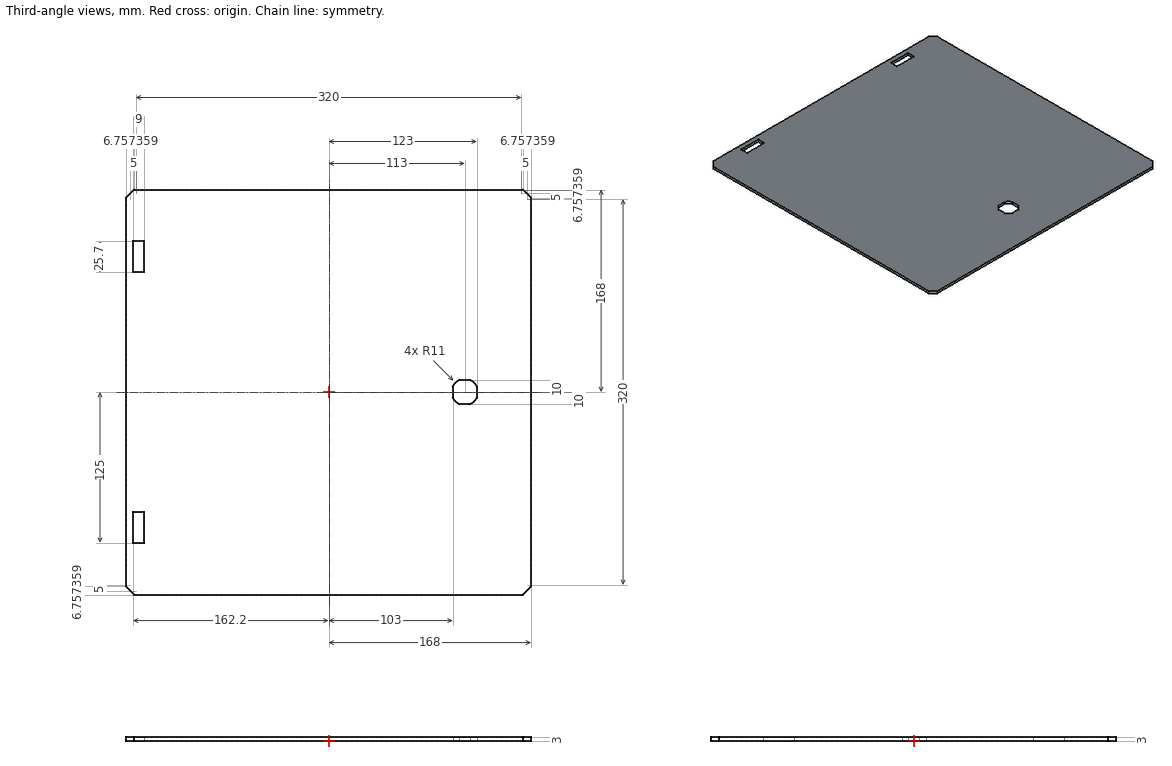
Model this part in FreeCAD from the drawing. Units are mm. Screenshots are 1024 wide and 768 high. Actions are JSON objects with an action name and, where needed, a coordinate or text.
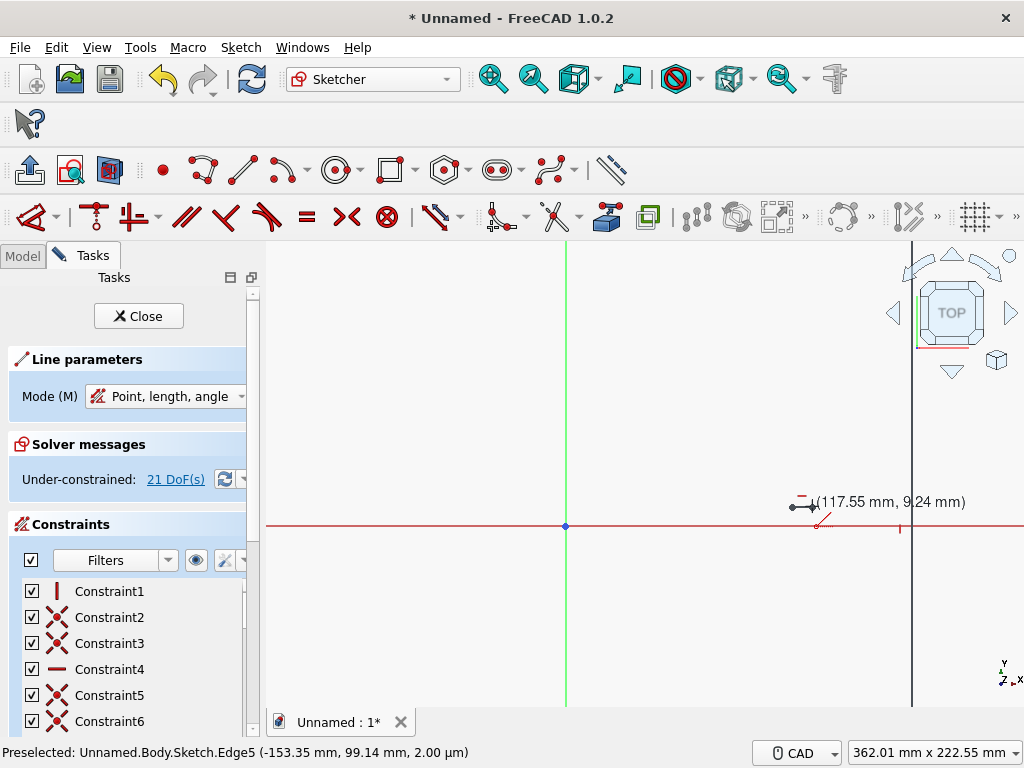
{"action": "scroll", "coordinate": [823, 517], "scroll_direction": "up", "scroll_amount": 3}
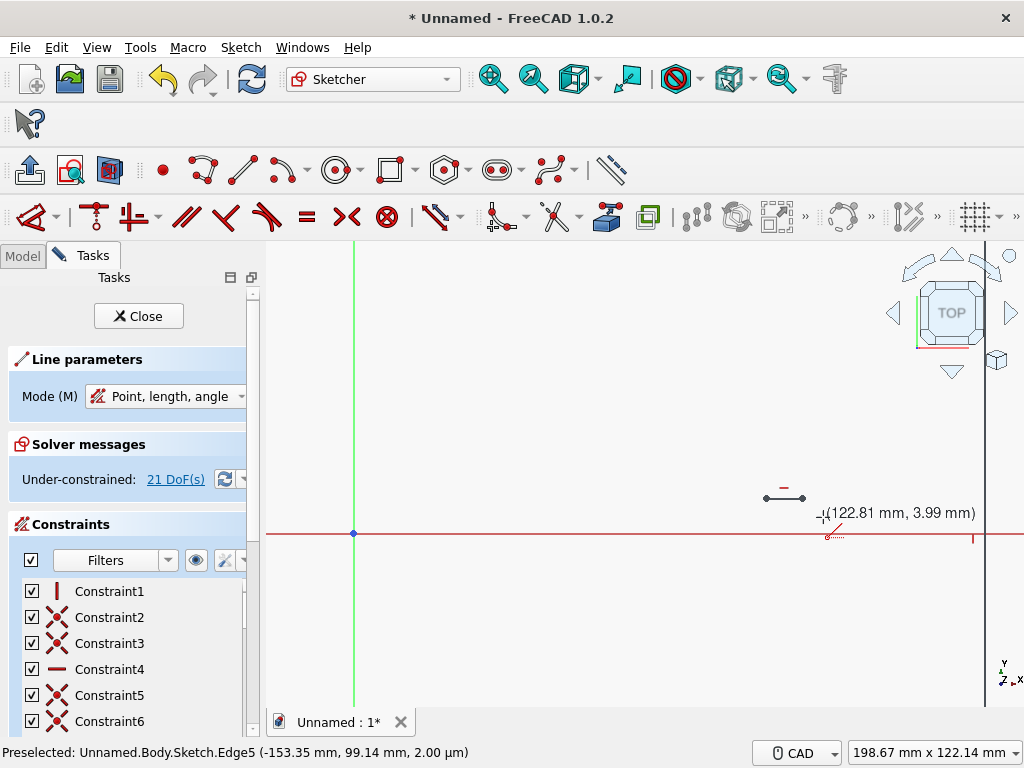
{"action": "left_click", "coordinate": [823, 516]}
{"action": "left_click", "coordinate": [823, 551]}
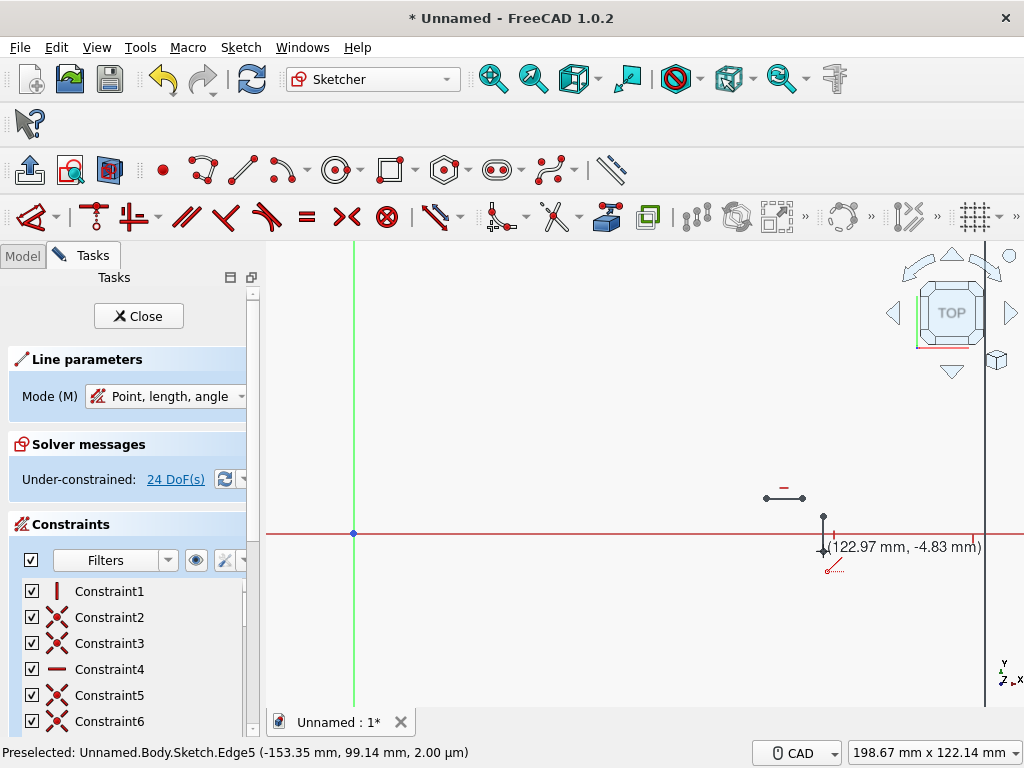
{"action": "left_click", "coordinate": [802, 572]}
{"action": "left_click", "coordinate": [767, 572]}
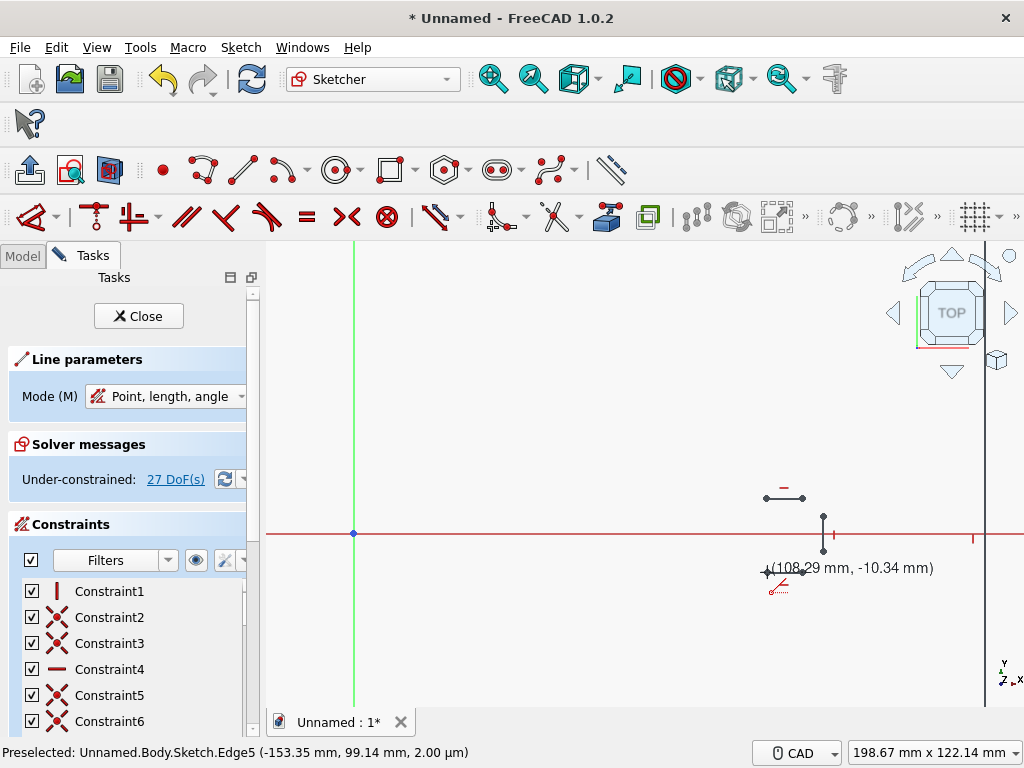
{"action": "left_click", "coordinate": [747, 551]}
{"action": "left_click", "coordinate": [747, 516]}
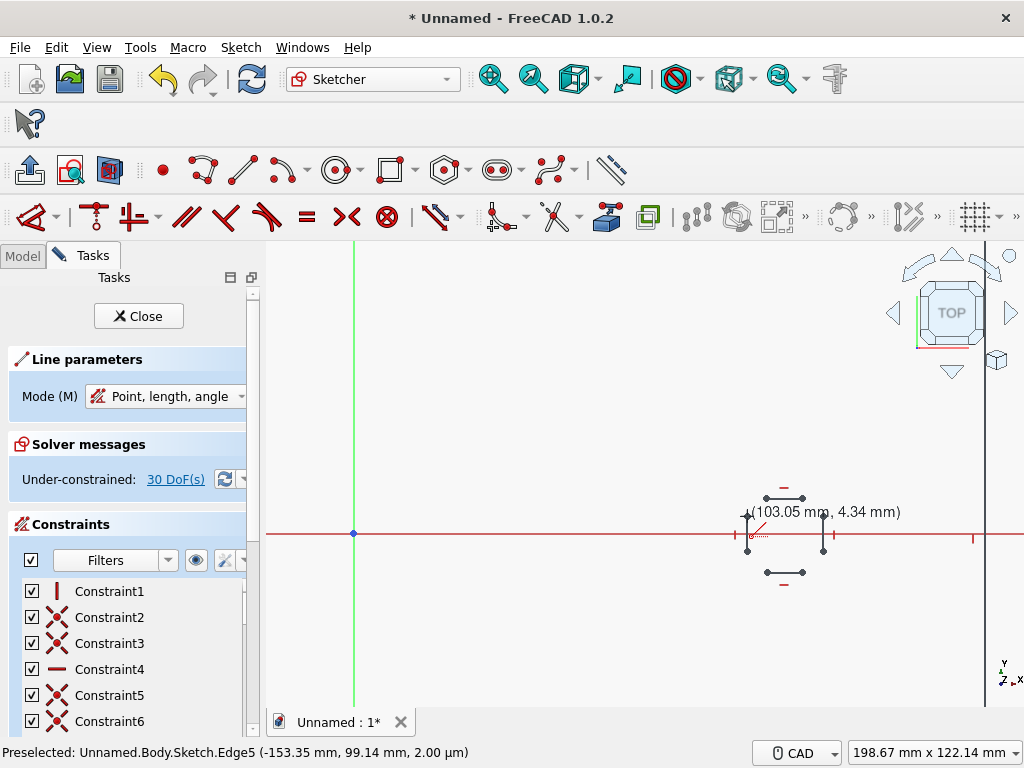
{"action": "left_click", "coordinate": [310, 170]}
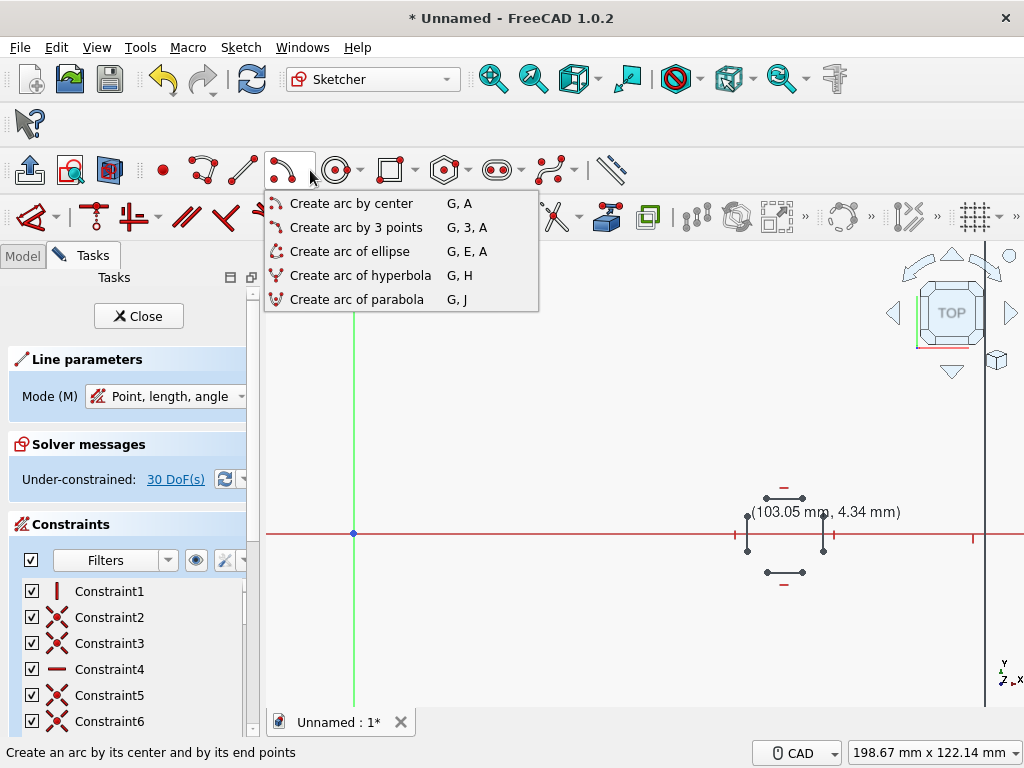
{"action": "left_click", "coordinate": [402, 227]}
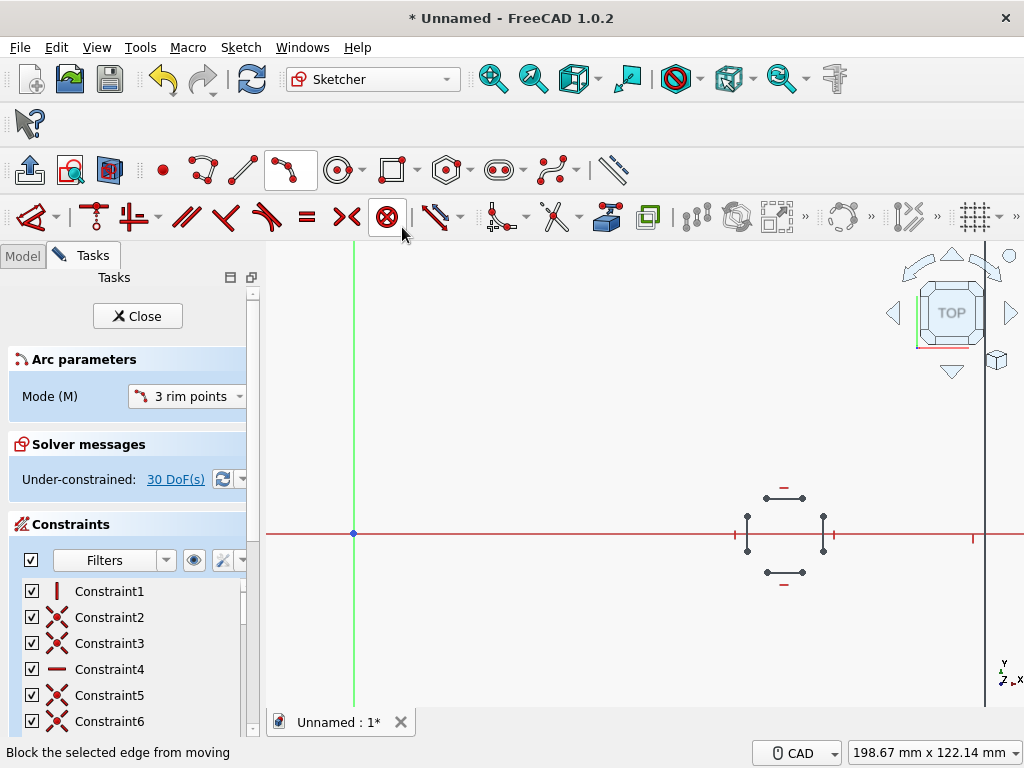
{"action": "left_click", "coordinate": [802, 499]}
{"action": "left_click", "coordinate": [823, 517]}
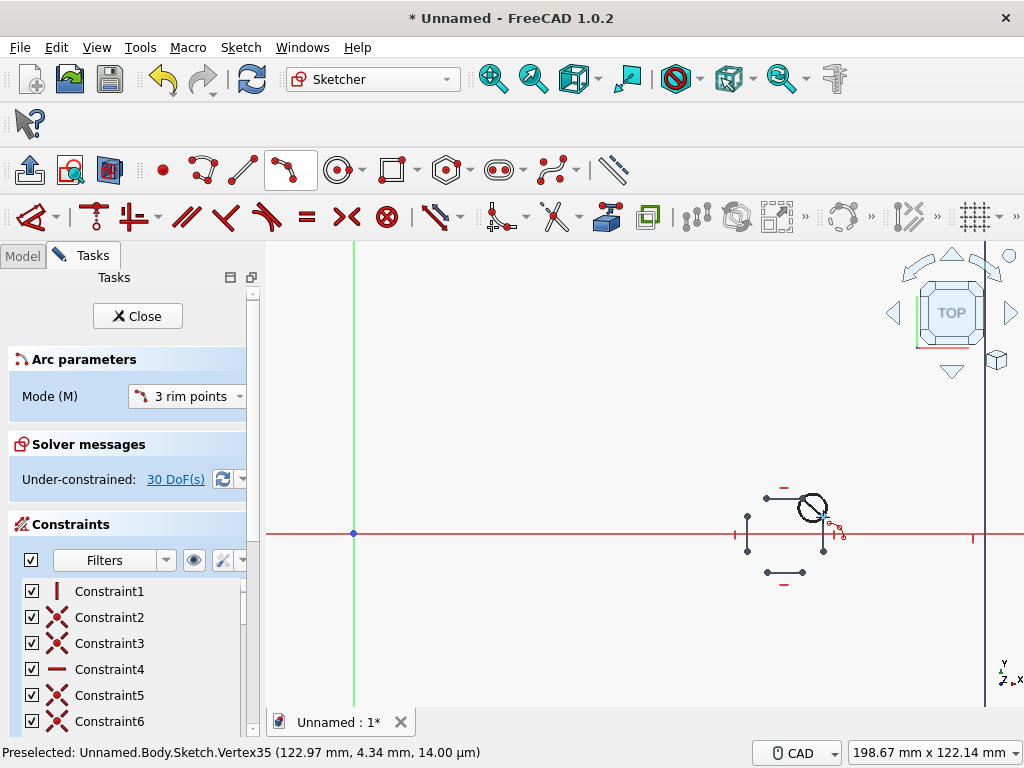
{"action": "scroll", "coordinate": [815, 504], "scroll_direction": "up", "scroll_amount": 9}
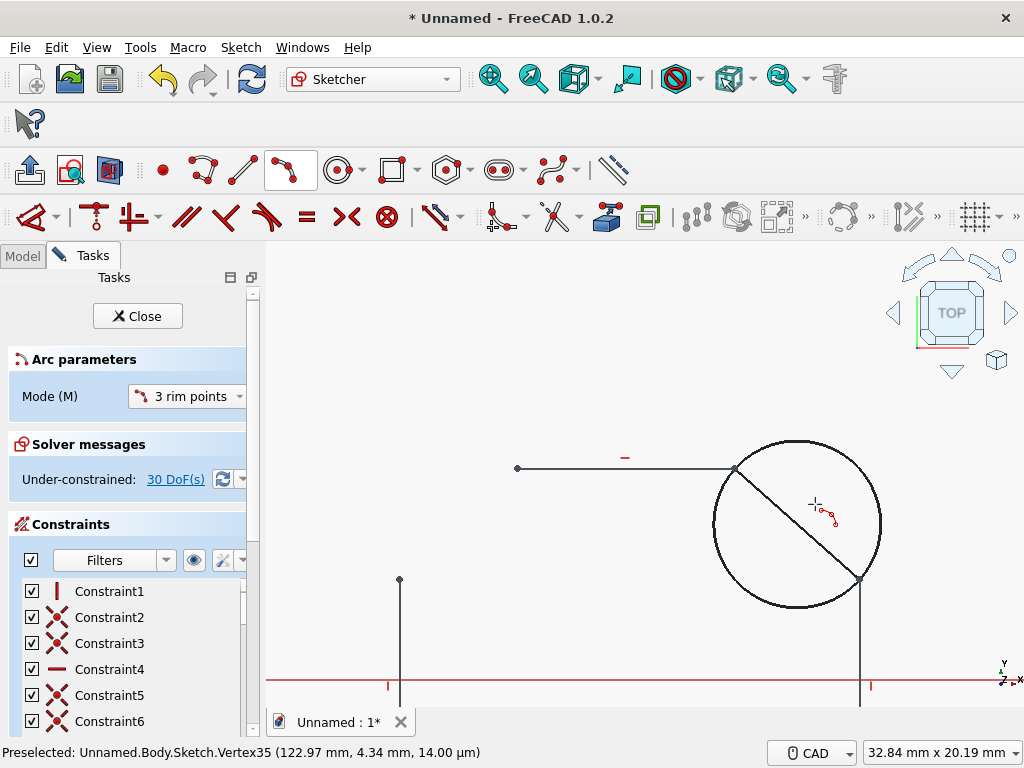
{"action": "left_click", "coordinate": [809, 500]}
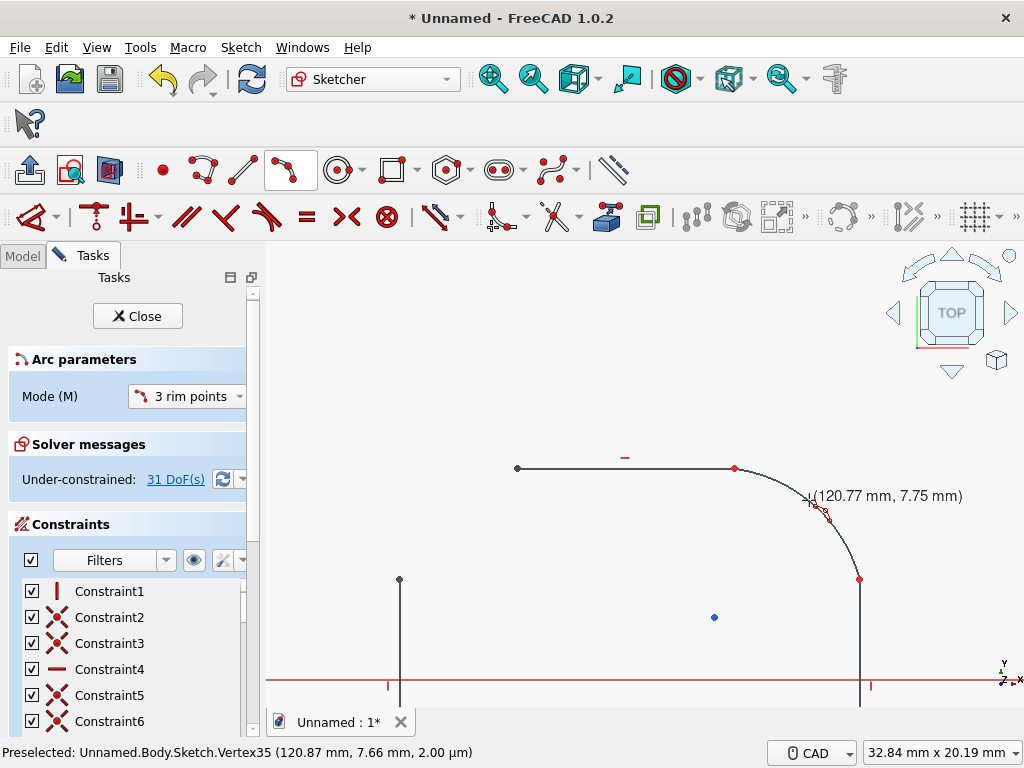
{"action": "scroll", "coordinate": [685, 465], "scroll_direction": "down", "scroll_amount": 16}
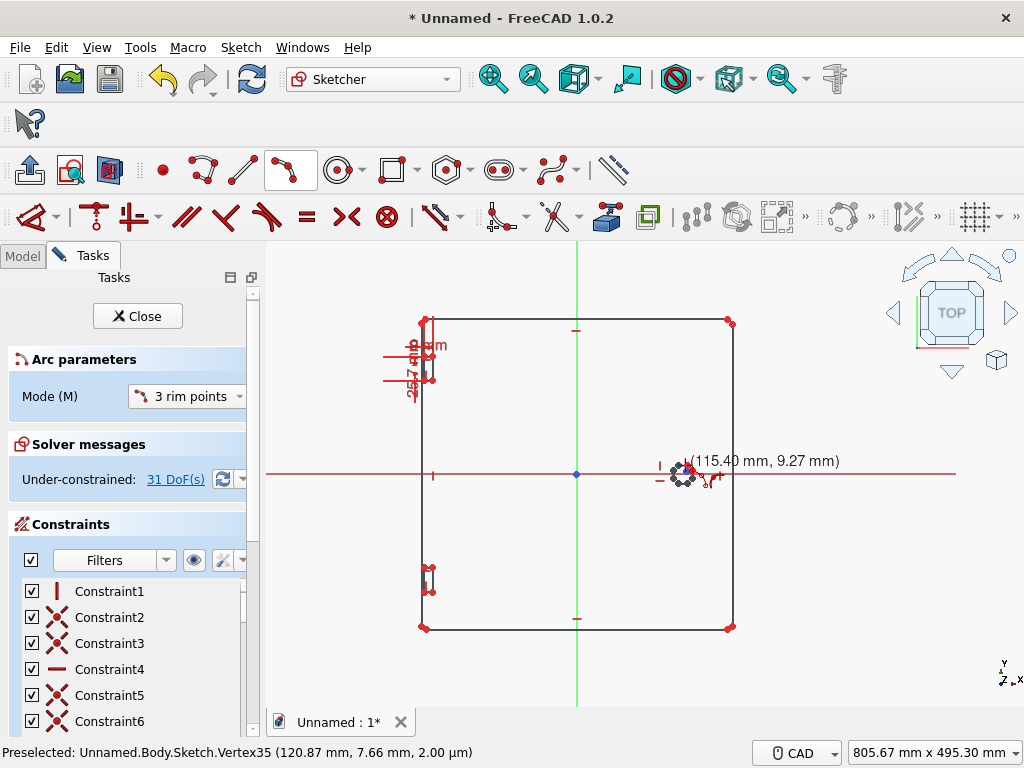
{"action": "scroll", "coordinate": [693, 479], "scroll_direction": "up", "scroll_amount": 7}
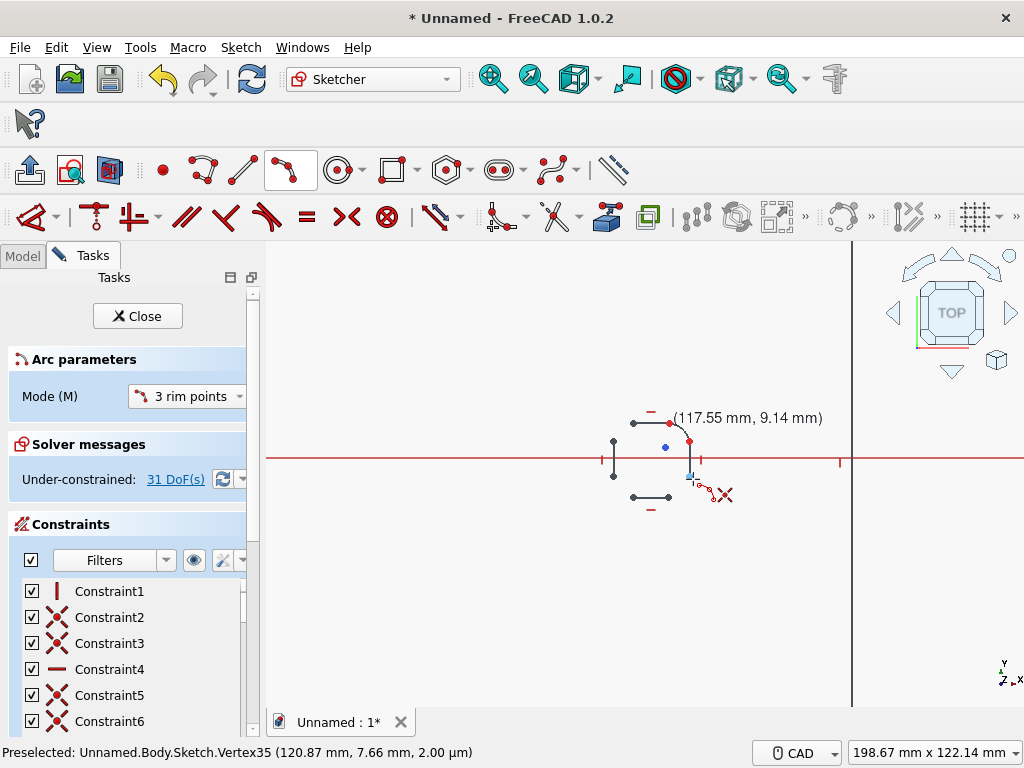
{"action": "left_click", "coordinate": [690, 477]}
{"action": "left_click", "coordinate": [669, 498]}